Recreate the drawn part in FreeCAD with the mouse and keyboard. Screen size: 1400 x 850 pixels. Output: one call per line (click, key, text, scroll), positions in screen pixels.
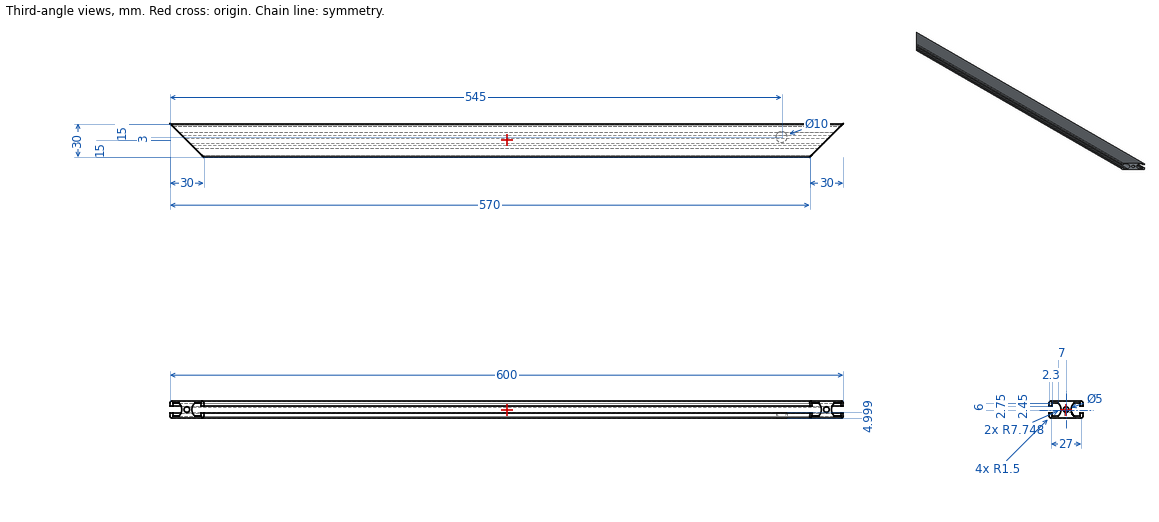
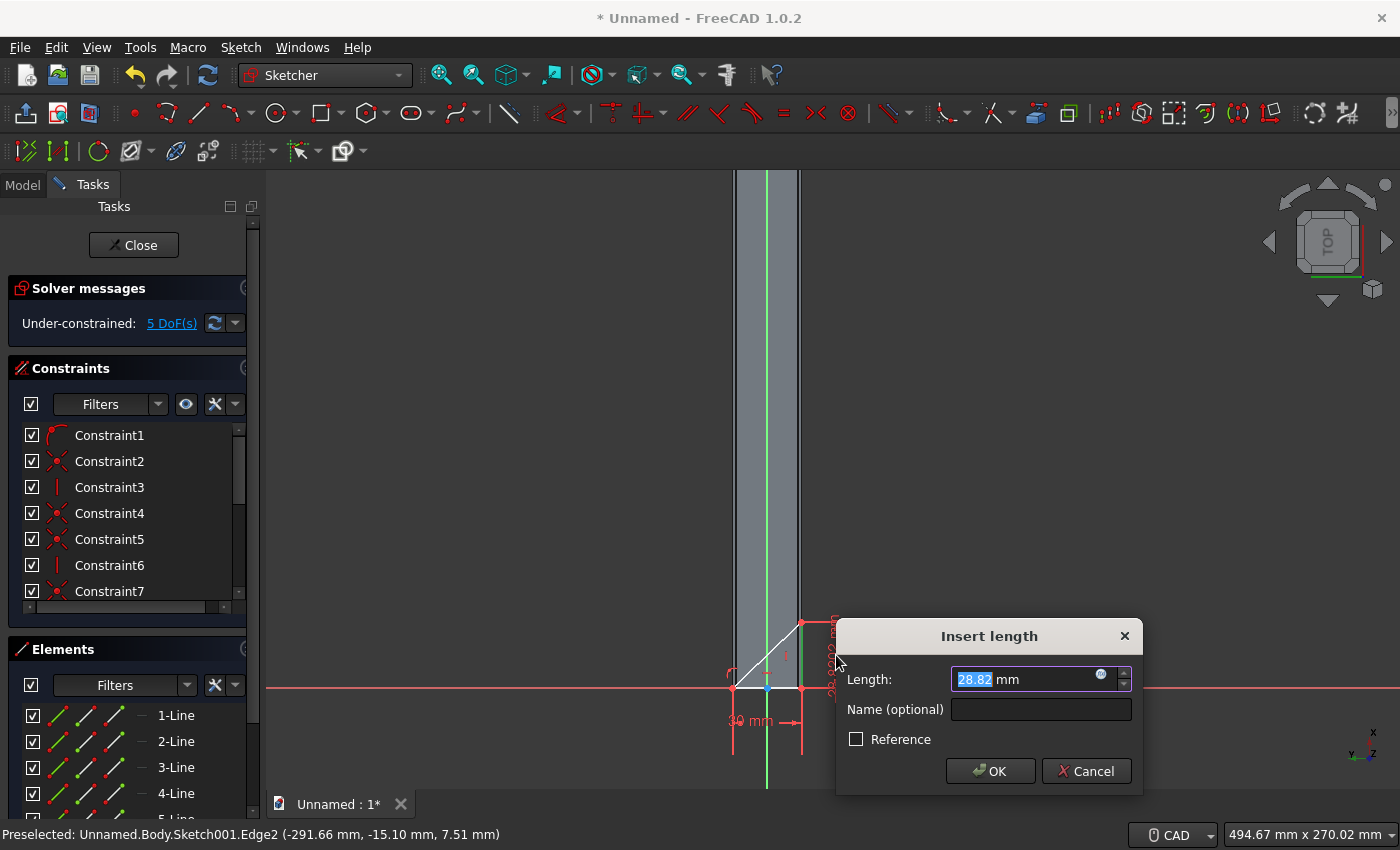
text(30)
key(Return)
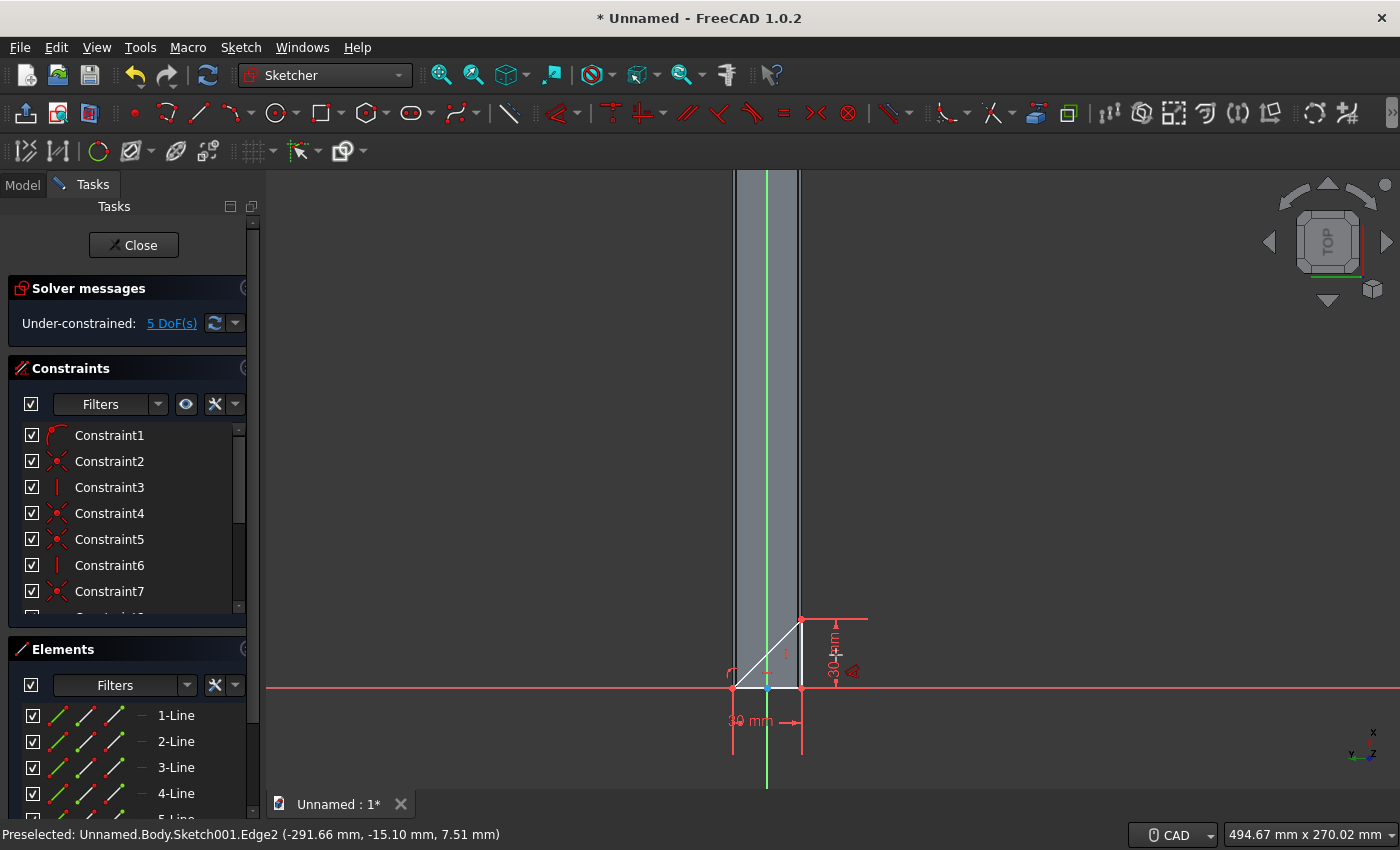
scroll(763, 686, down, 6)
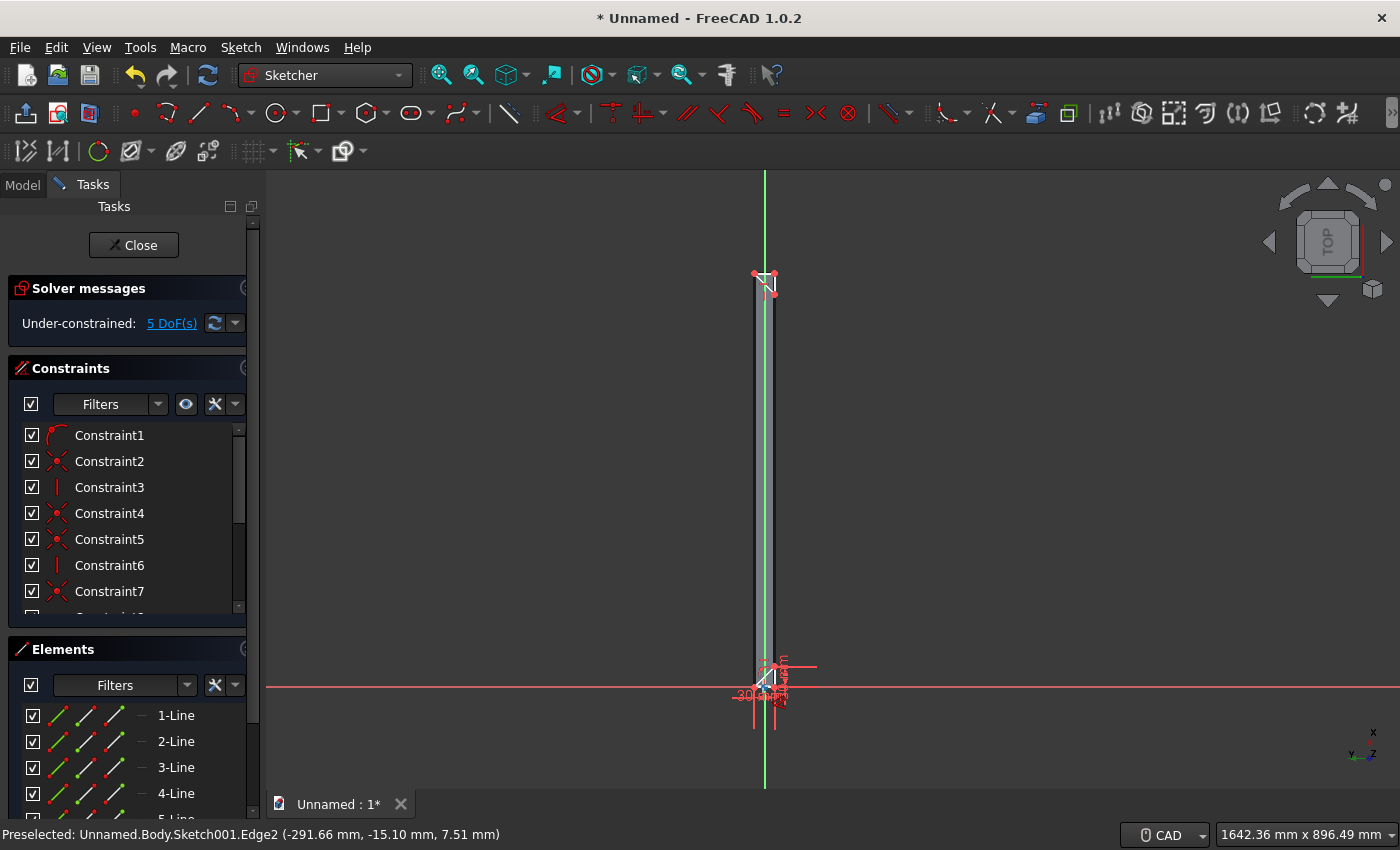
scroll(775, 288, up, 6)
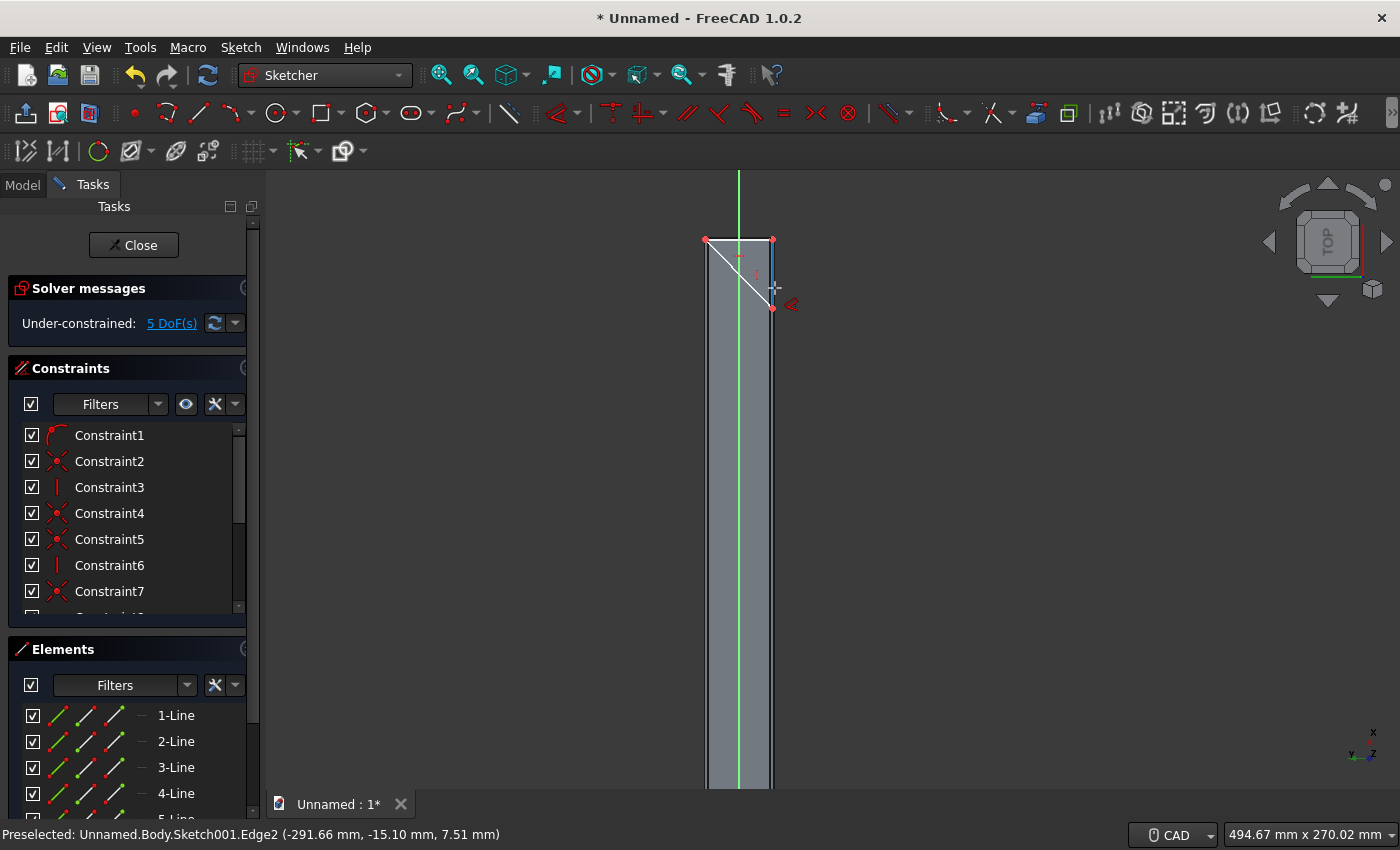
click(773, 288)
click(807, 274)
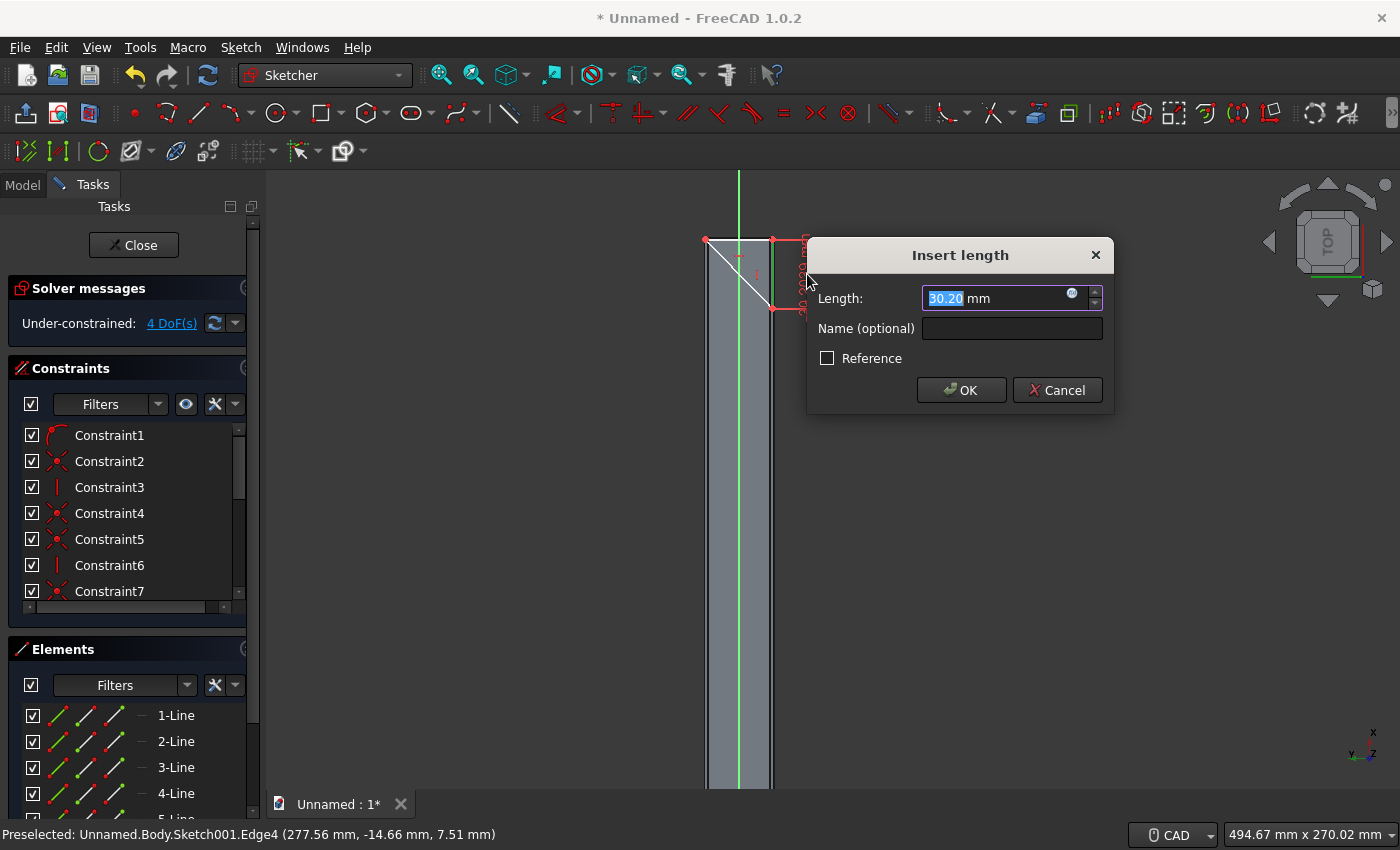
text(30)
key(Return)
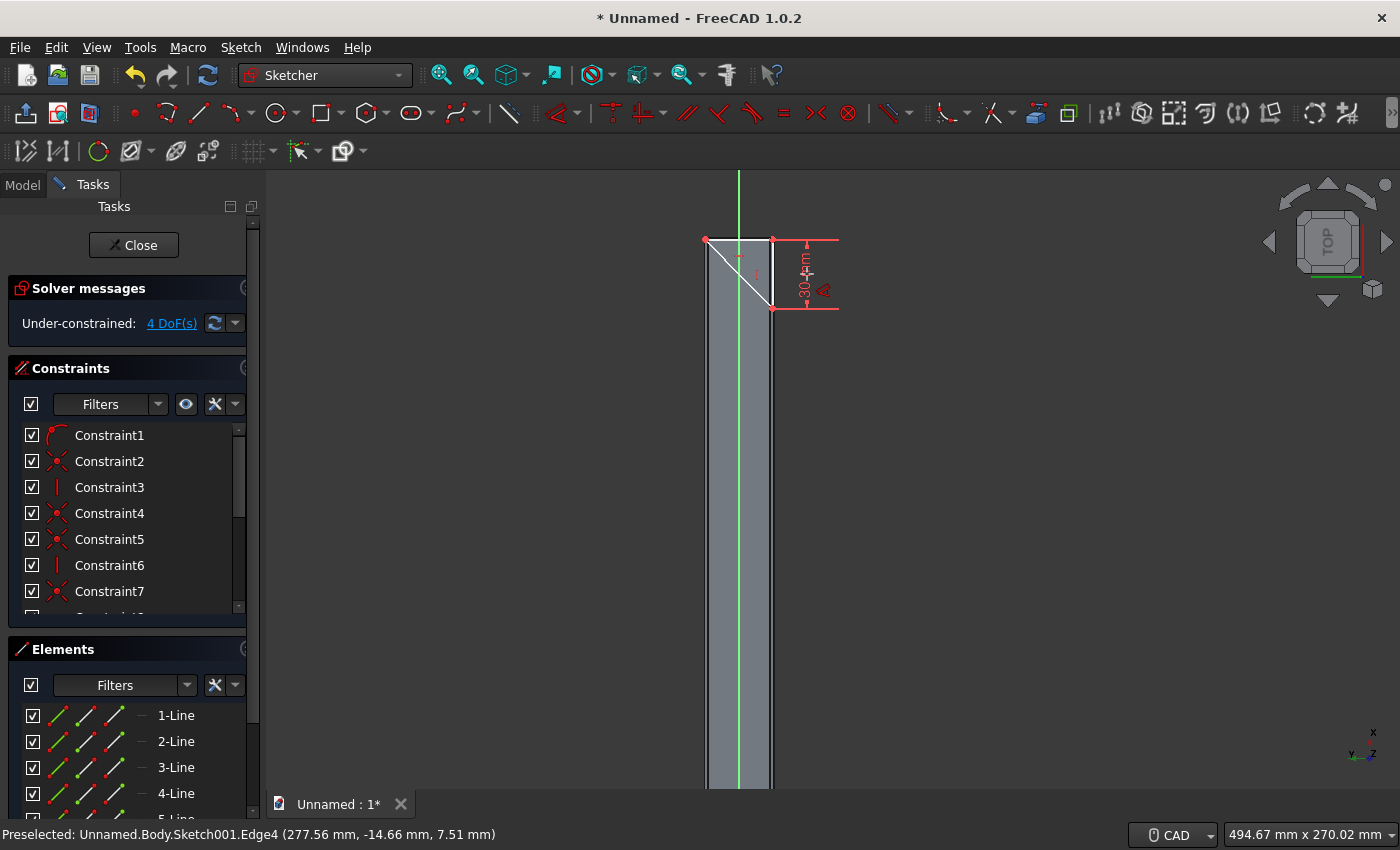
click(753, 240)
click(724, 206)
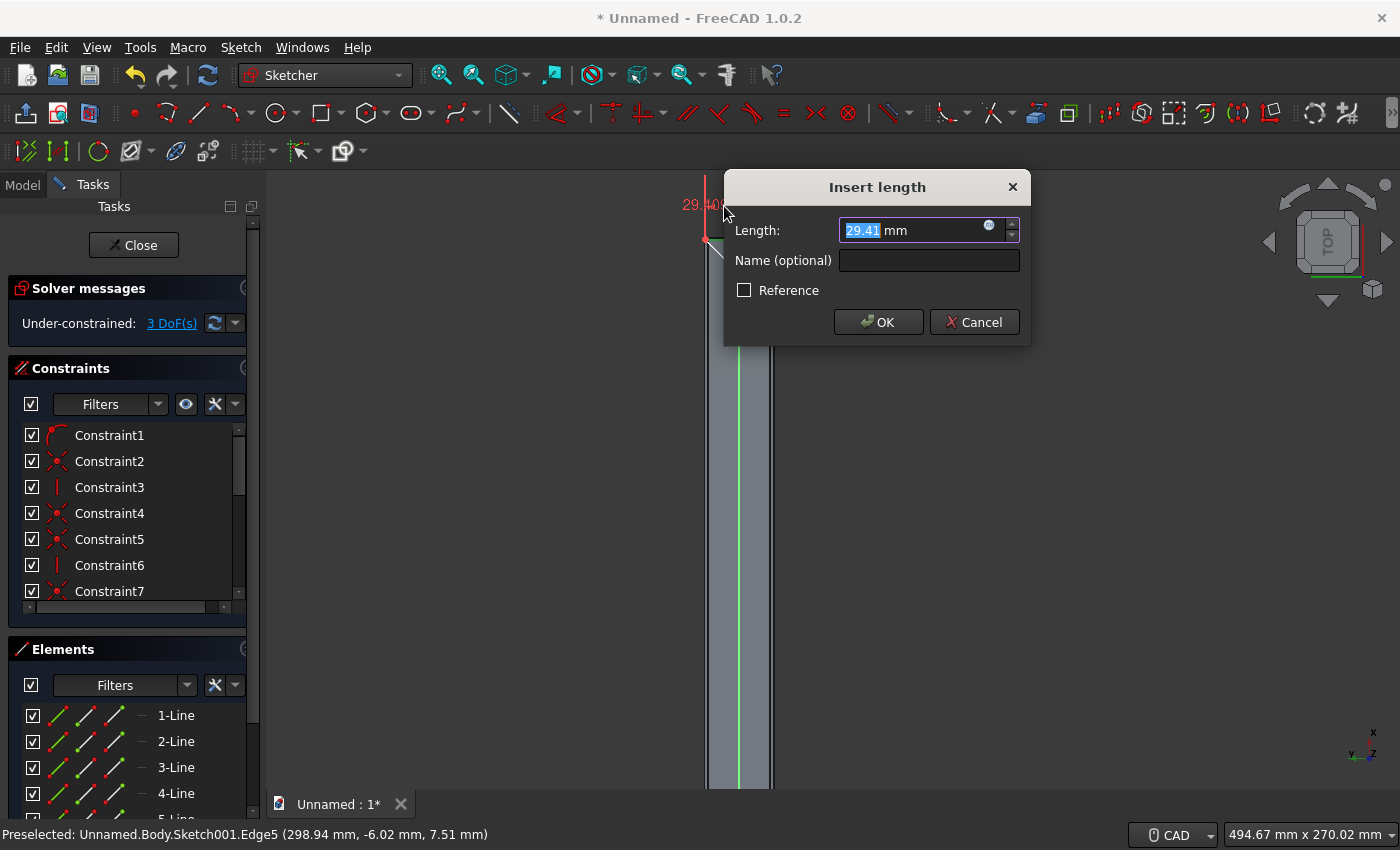
text(30)
key(Return)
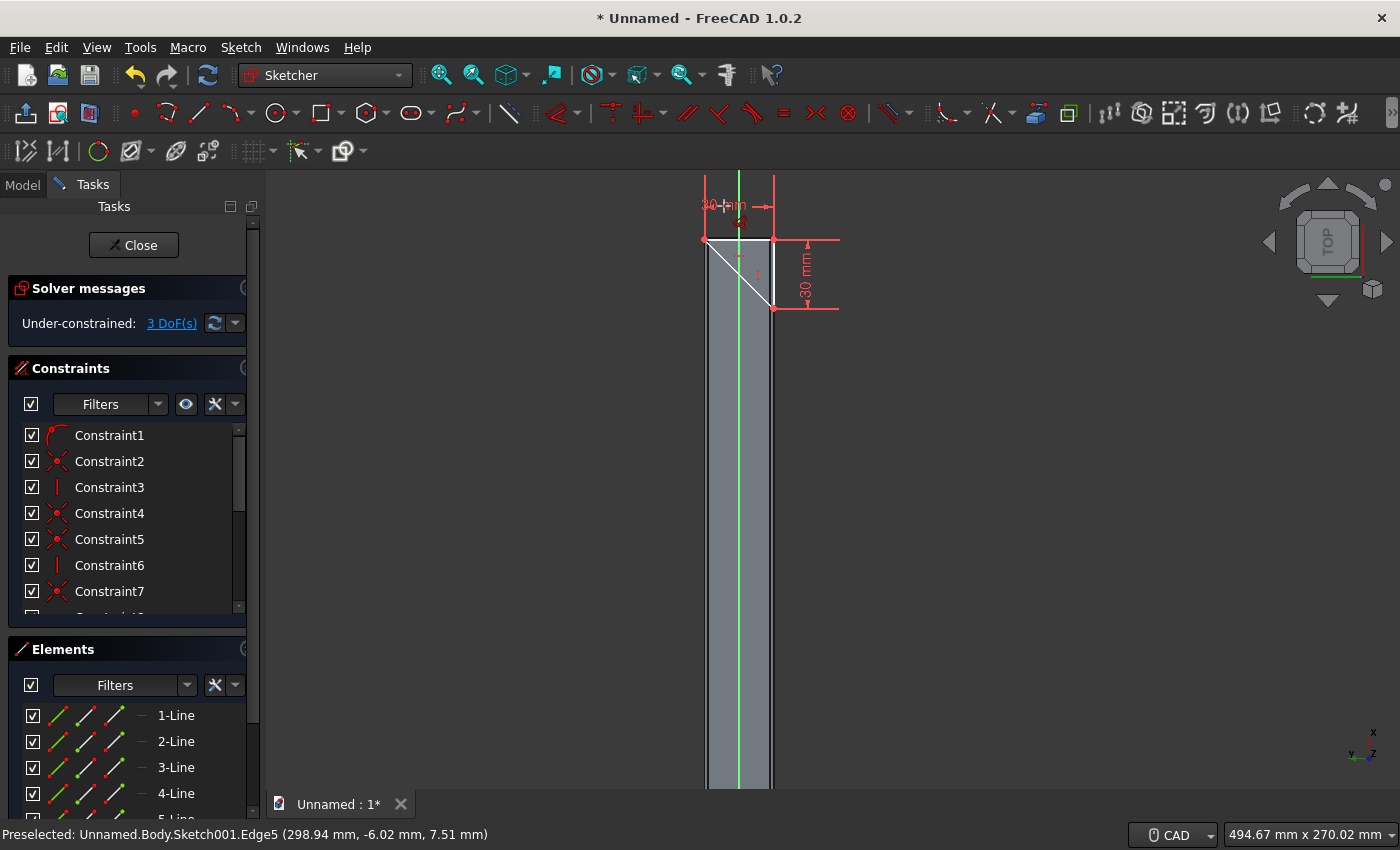
scroll(775, 287, down, 6)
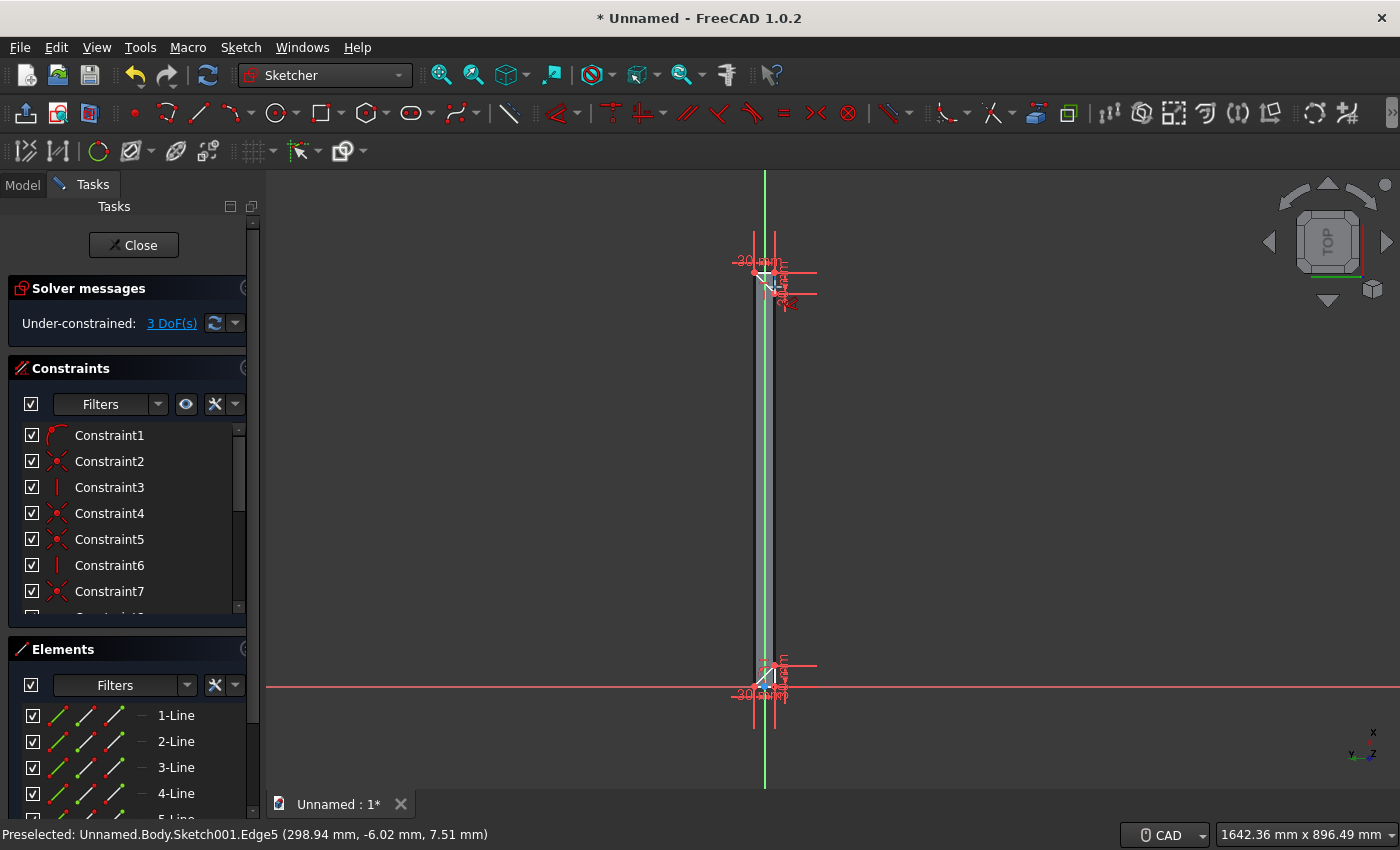
scroll(754, 687, up, 7)